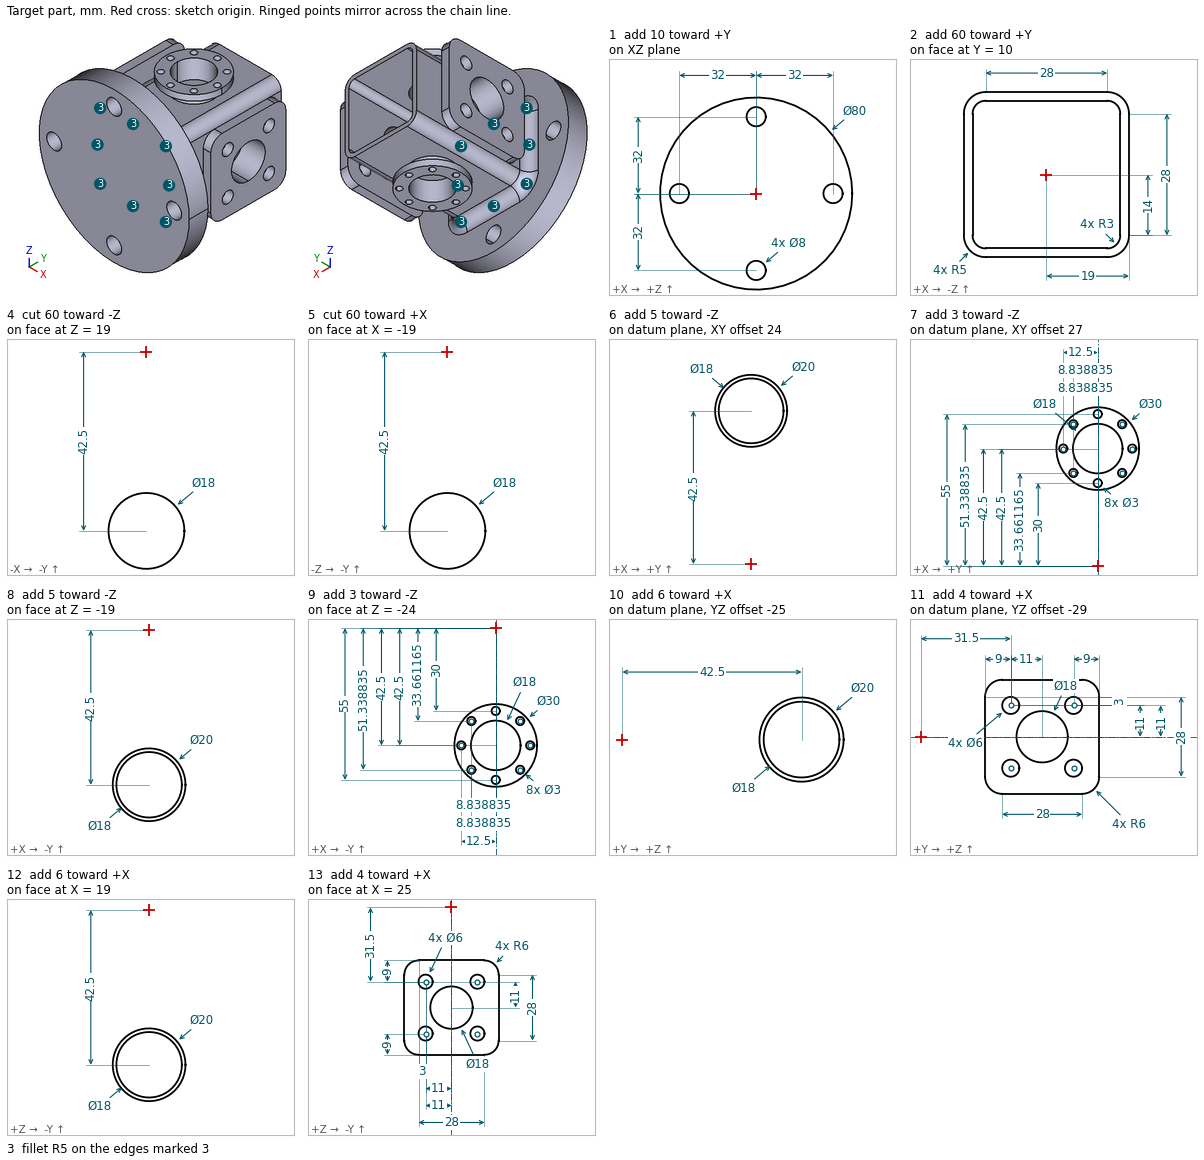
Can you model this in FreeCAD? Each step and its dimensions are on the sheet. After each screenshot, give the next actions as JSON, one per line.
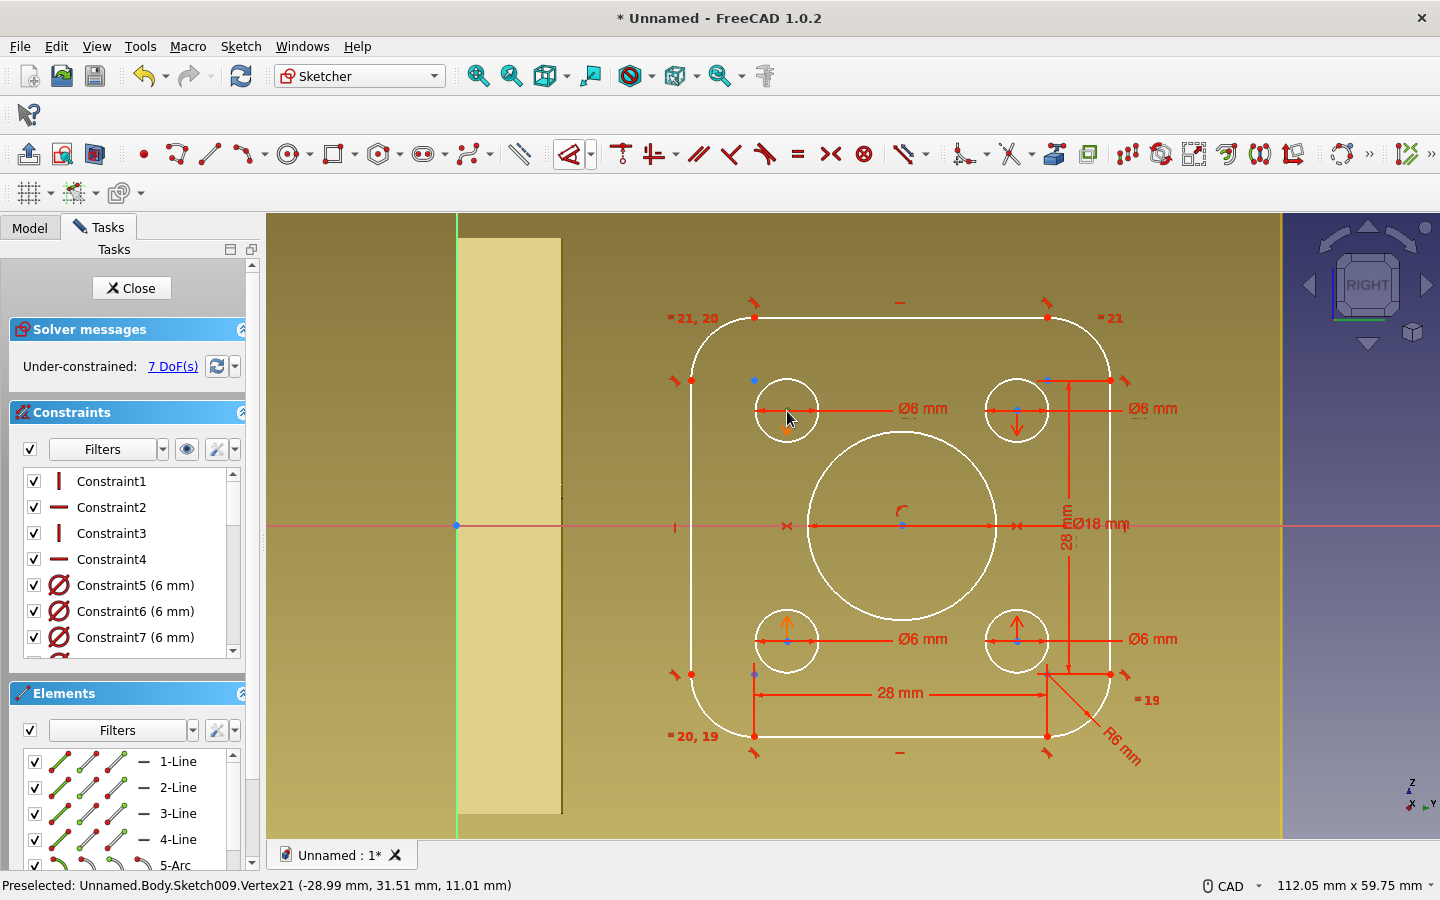
{"action": "key", "text": "i"}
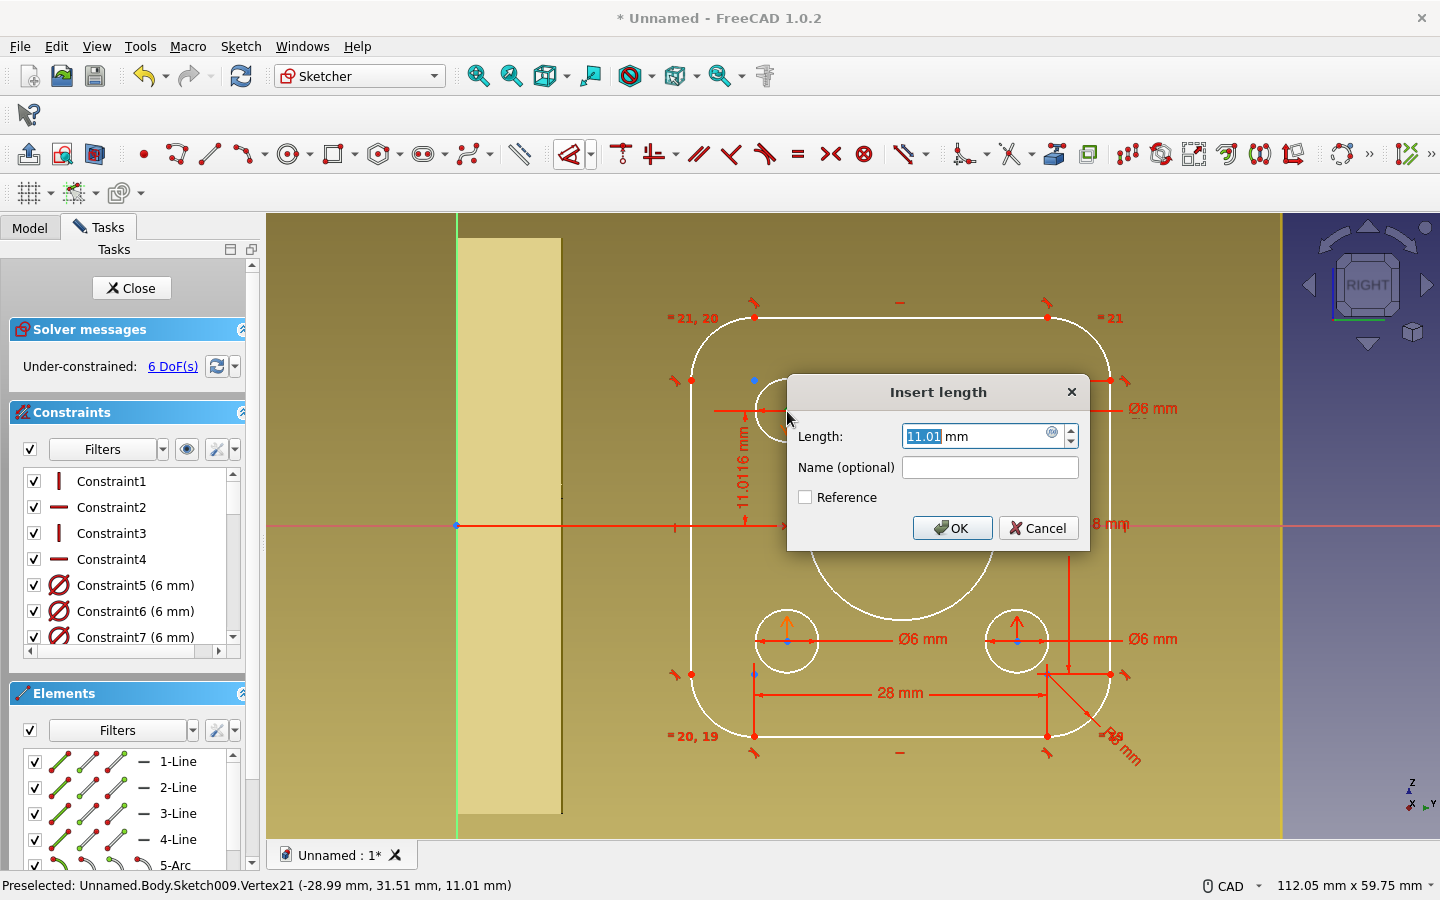
{"action": "type", "text": "11"}
{"action": "key", "text": "Return"}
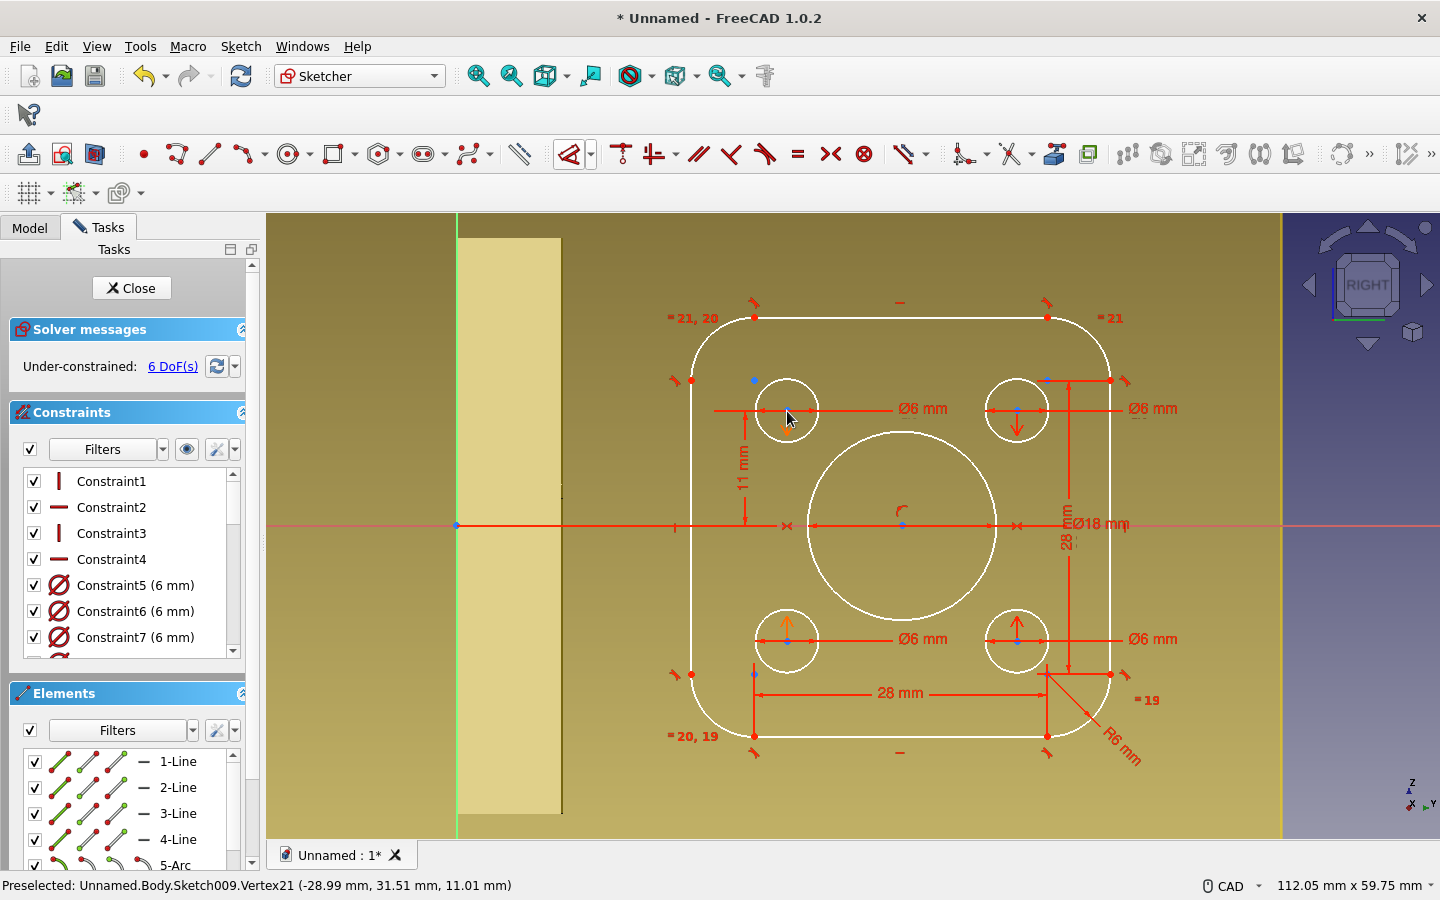
{"action": "left_click", "coordinate": [1017, 411]}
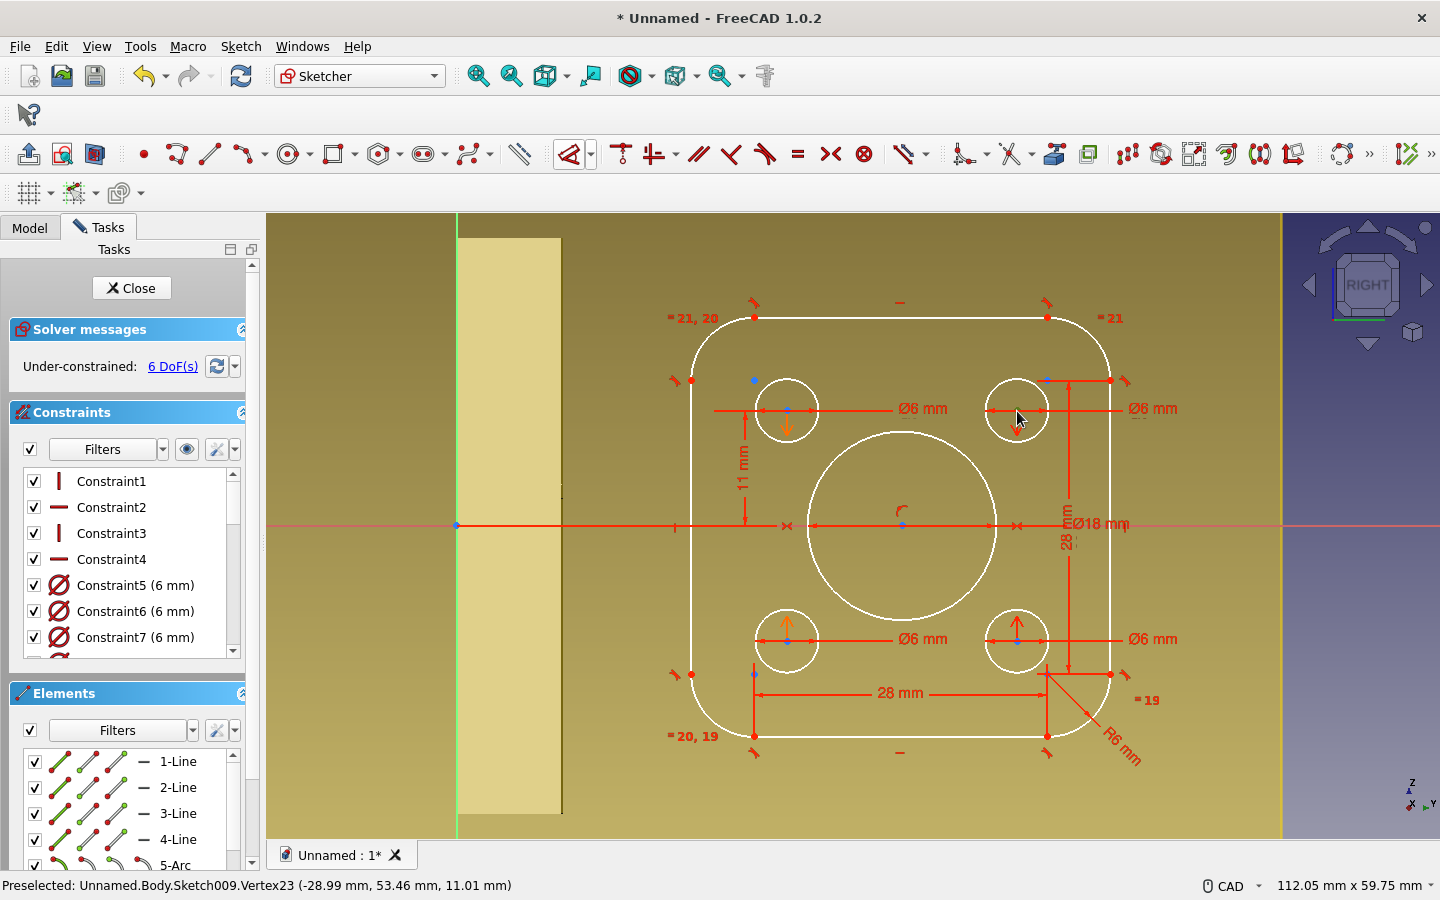
{"action": "left_click", "coordinate": [590, 154]}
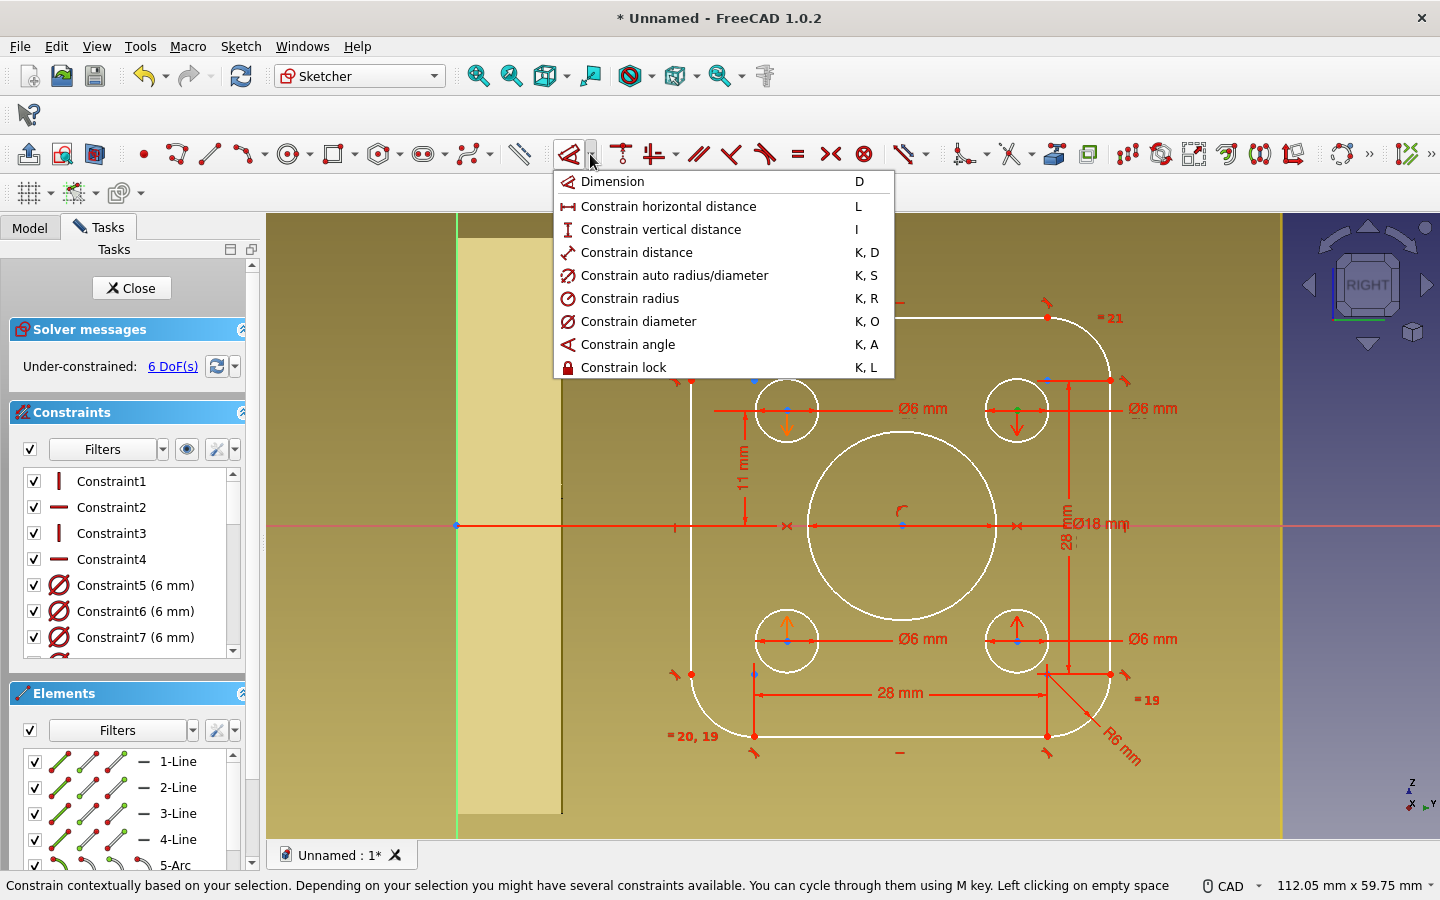
{"action": "left_click", "coordinate": [724, 230]}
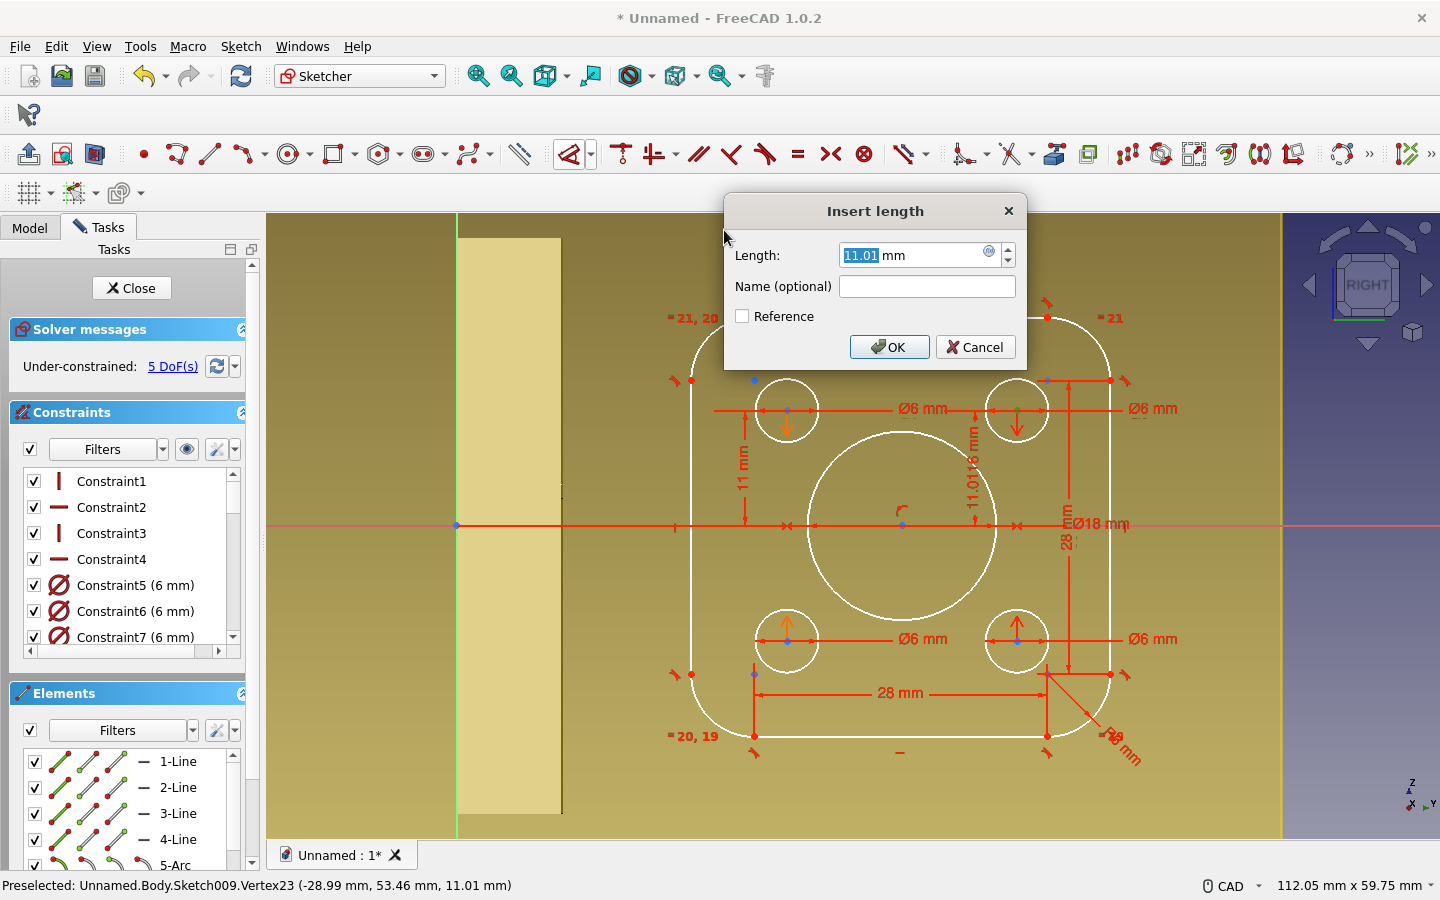
{"action": "type", "text": "11"}
{"action": "key", "text": "Return"}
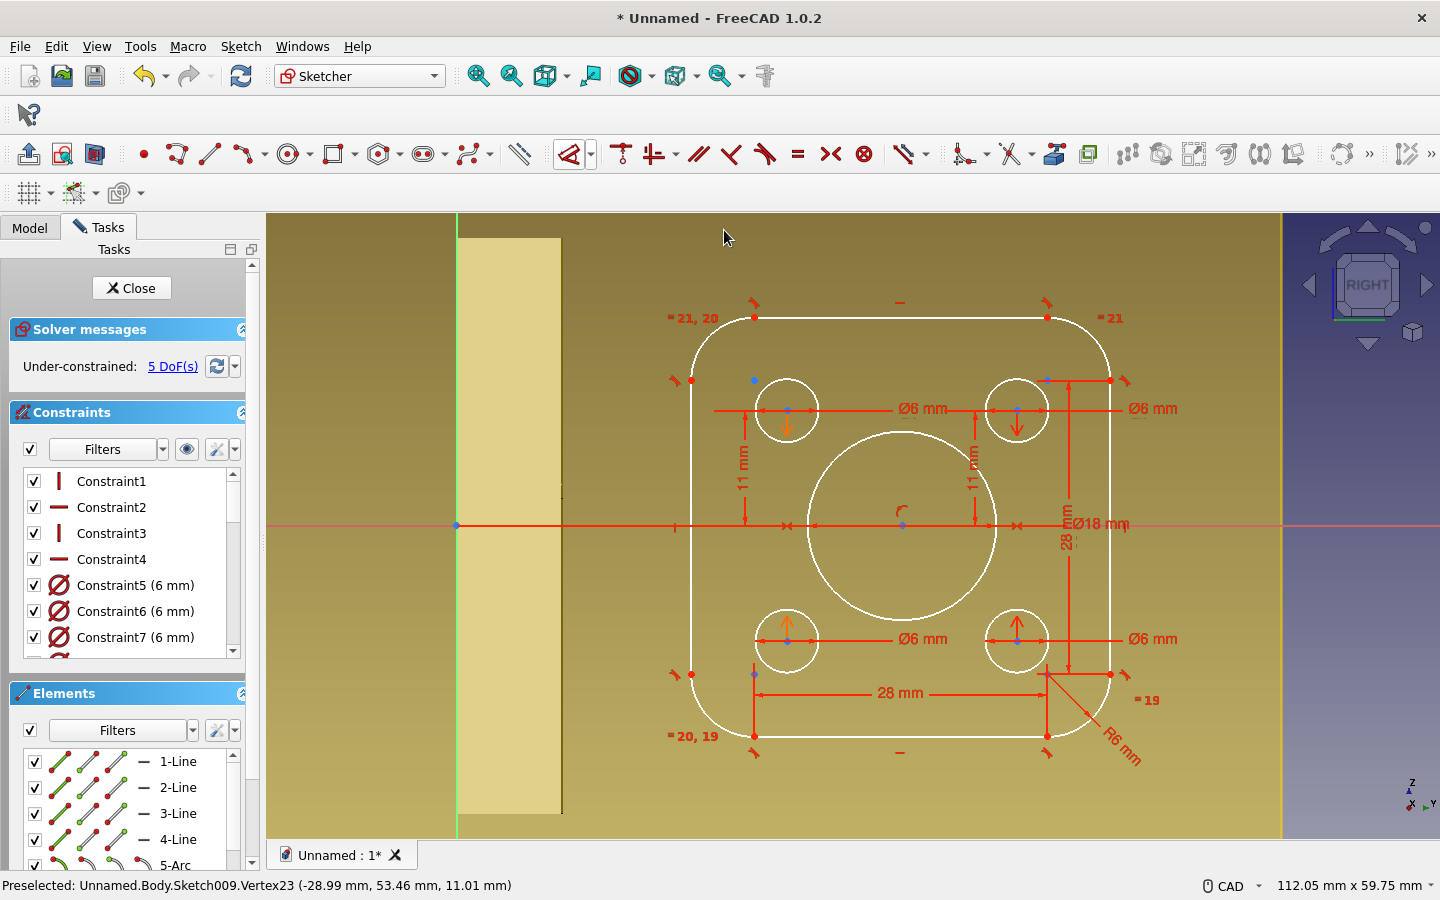
{"action": "left_click", "coordinate": [691, 381]}